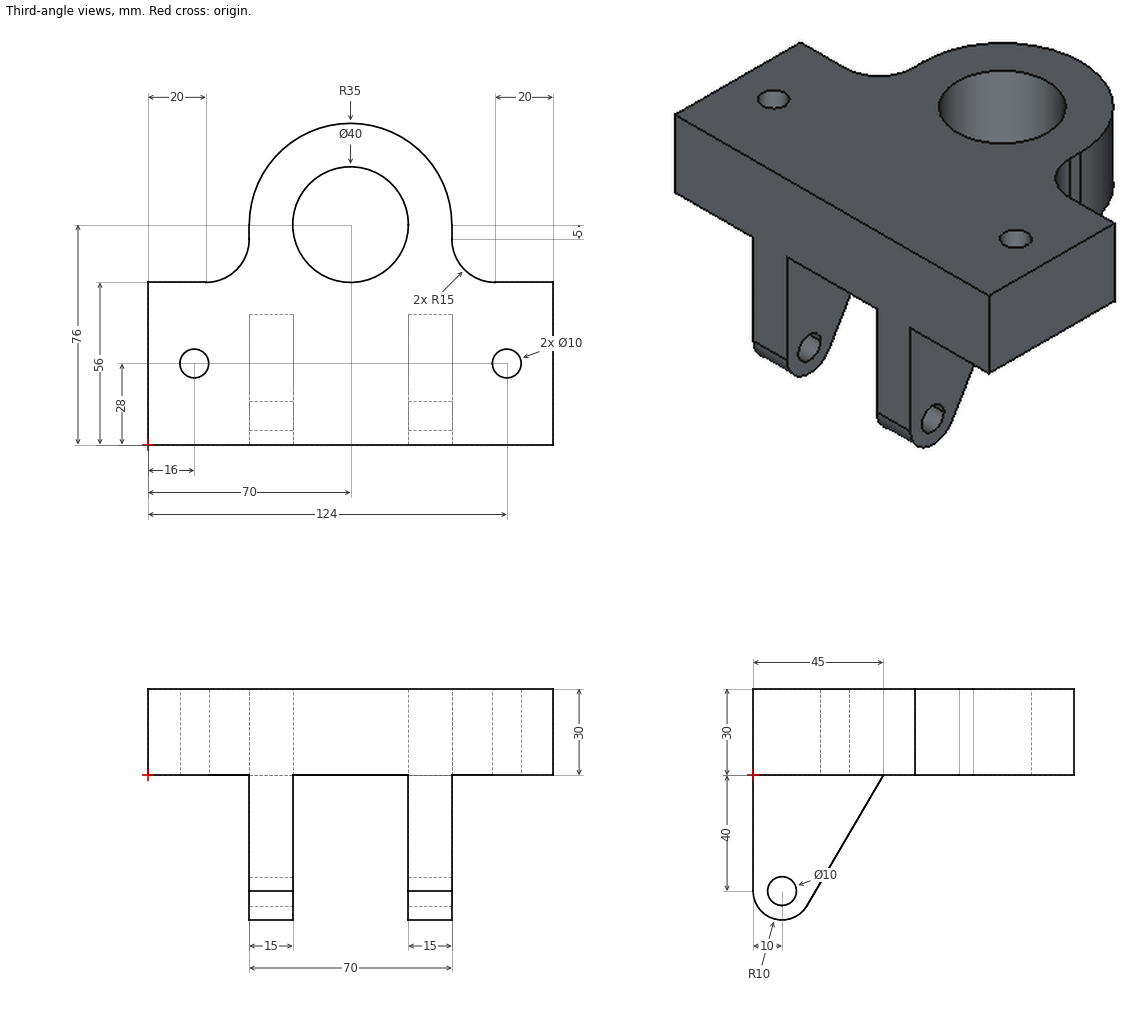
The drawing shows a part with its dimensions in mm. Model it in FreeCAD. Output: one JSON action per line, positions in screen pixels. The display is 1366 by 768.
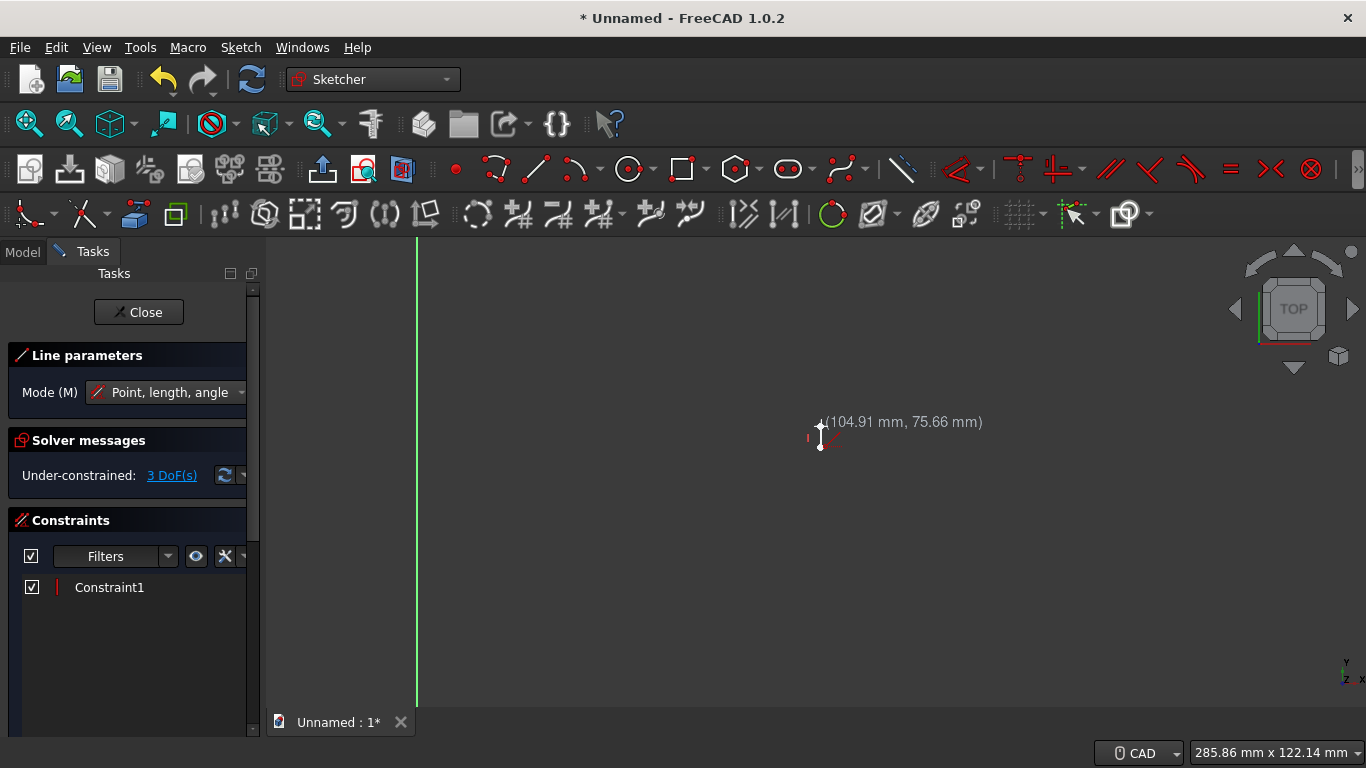
{"action": "left_click", "coordinate": [552, 426]}
{"action": "left_click", "coordinate": [552, 445]}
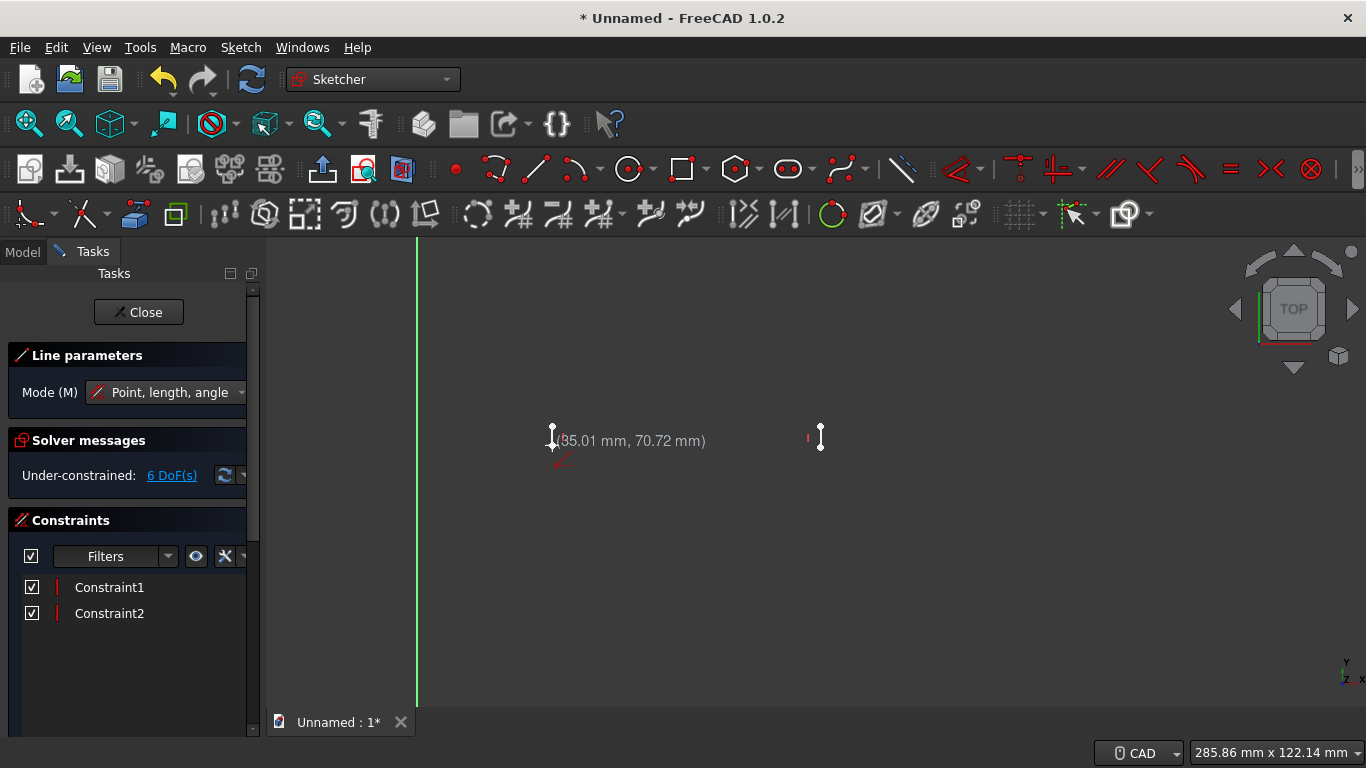
{"action": "left_click", "coordinate": [496, 170]}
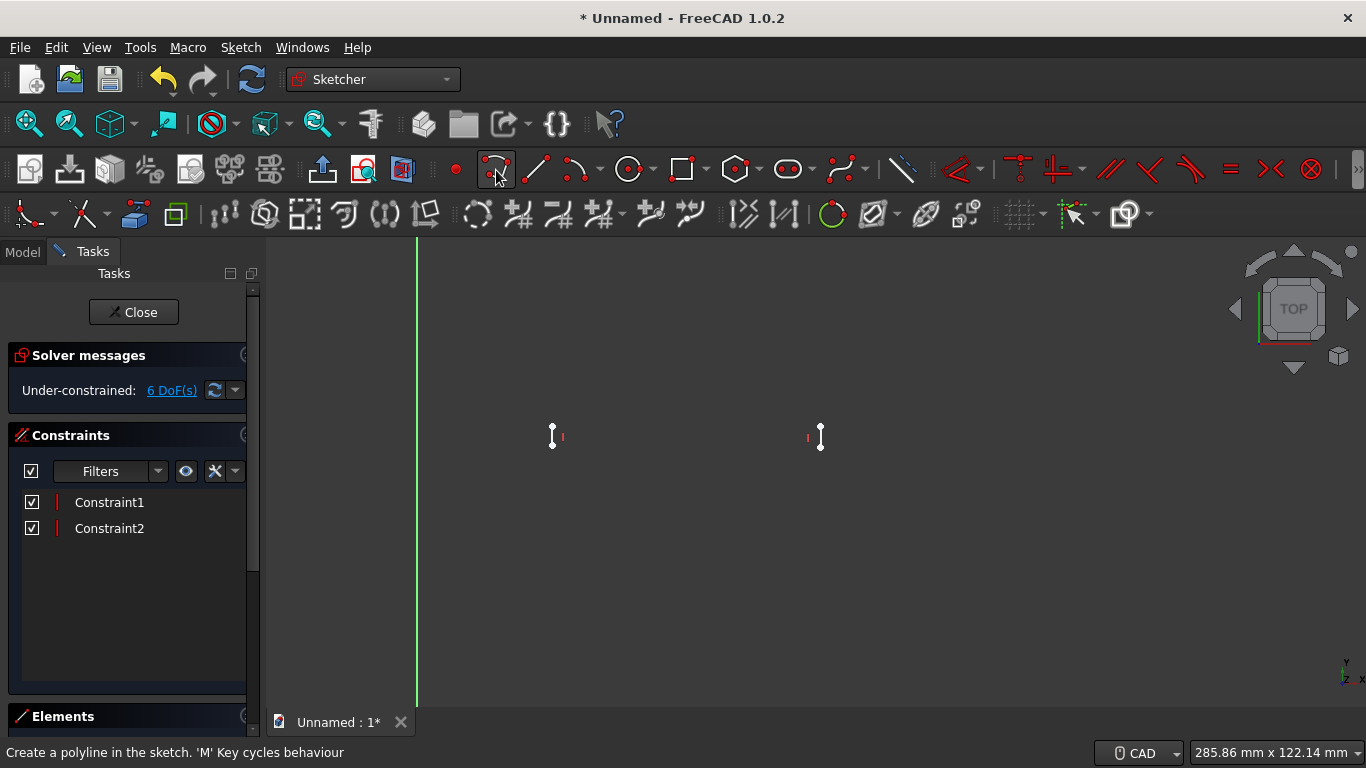
{"action": "left_click", "coordinate": [494, 503]}
{"action": "left_click", "coordinate": [417, 503]}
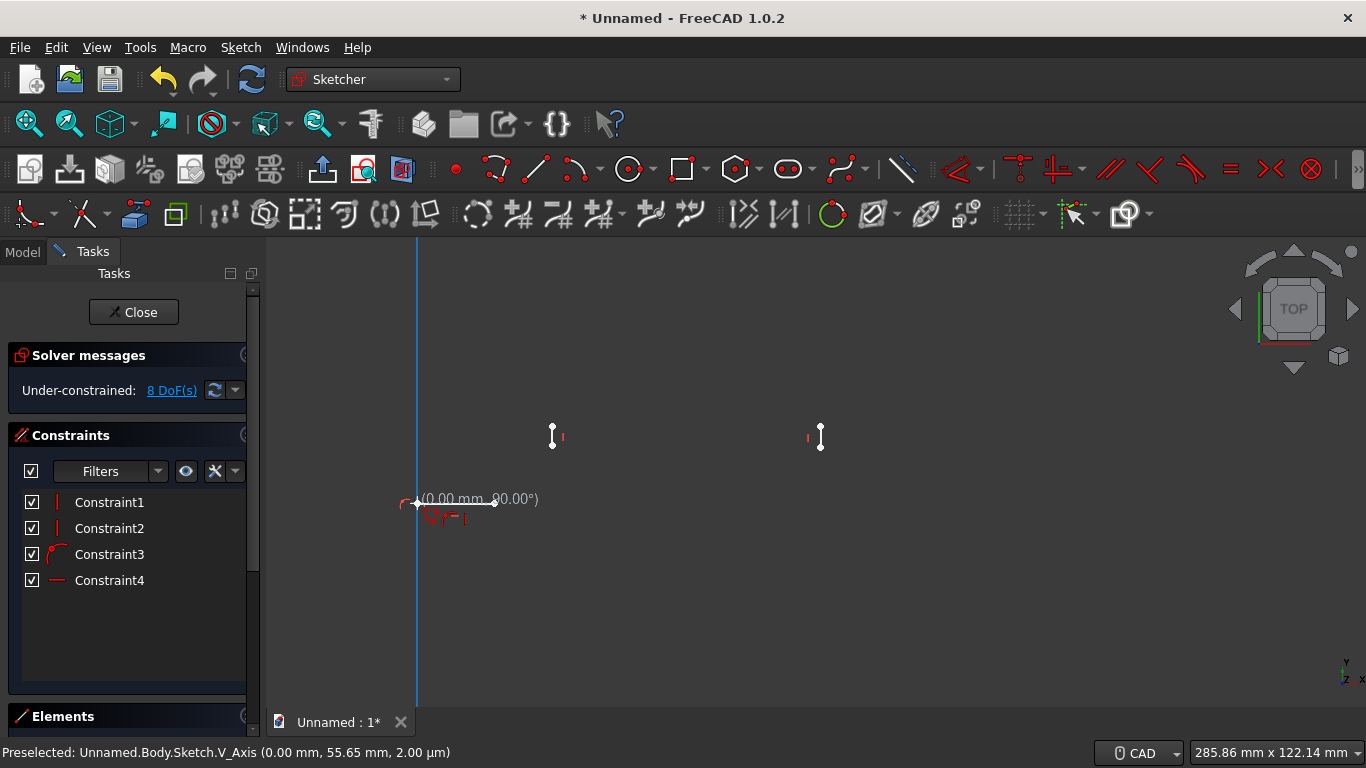
{"action": "scroll", "coordinate": [871, 406], "scroll_direction": "down", "scroll_amount": 2}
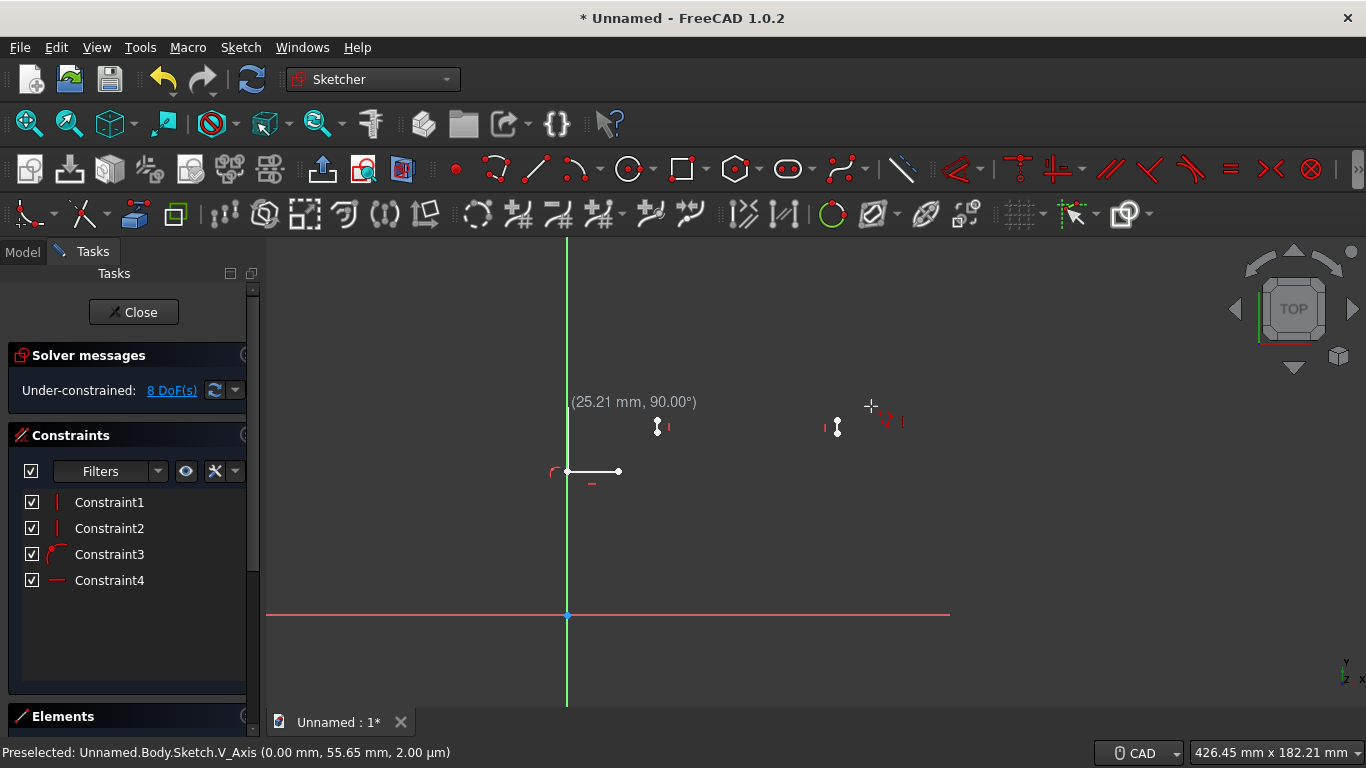
{"action": "left_click", "coordinate": [567, 615]}
{"action": "left_click", "coordinate": [928, 606]}
{"action": "left_click", "coordinate": [928, 471]}
{"action": "left_click", "coordinate": [877, 471]}
{"action": "right_click", "coordinate": [877, 471]}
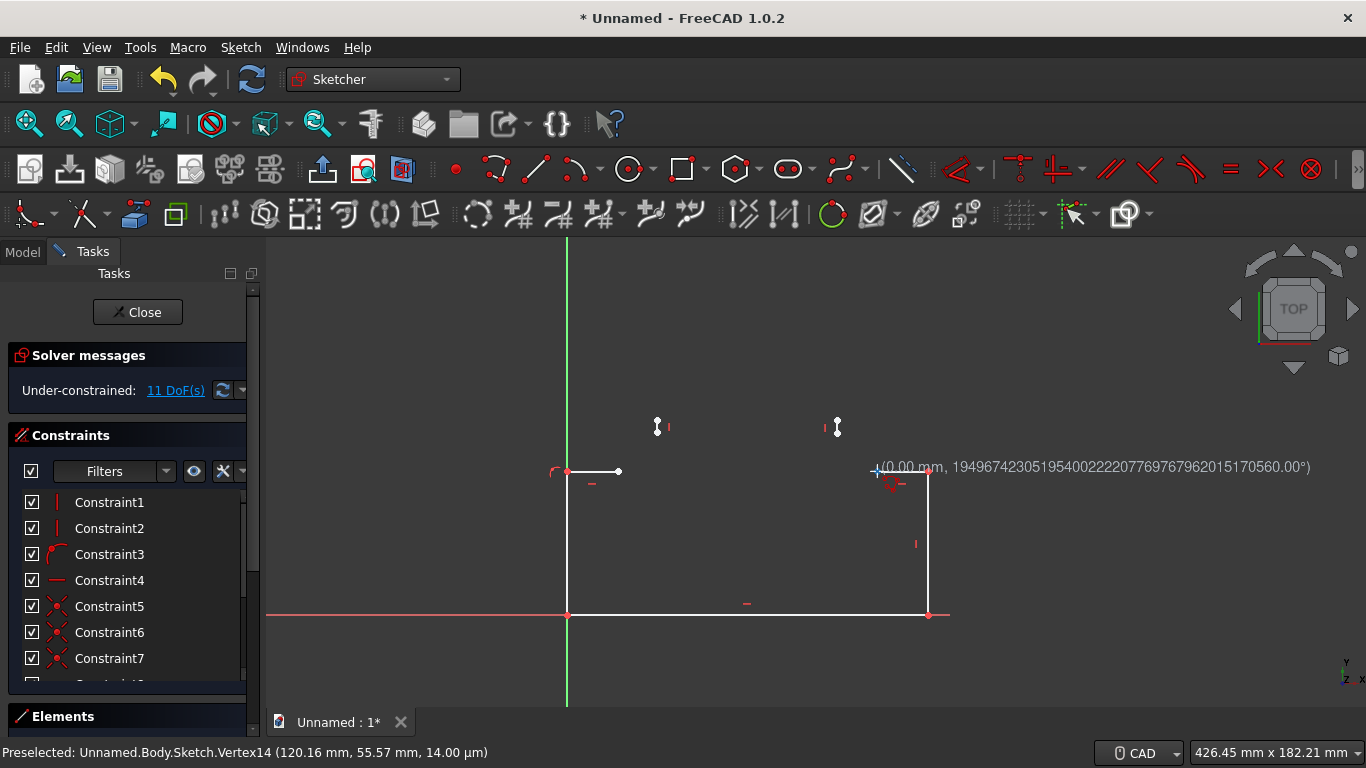
{"action": "key", "text": "g 3 a"}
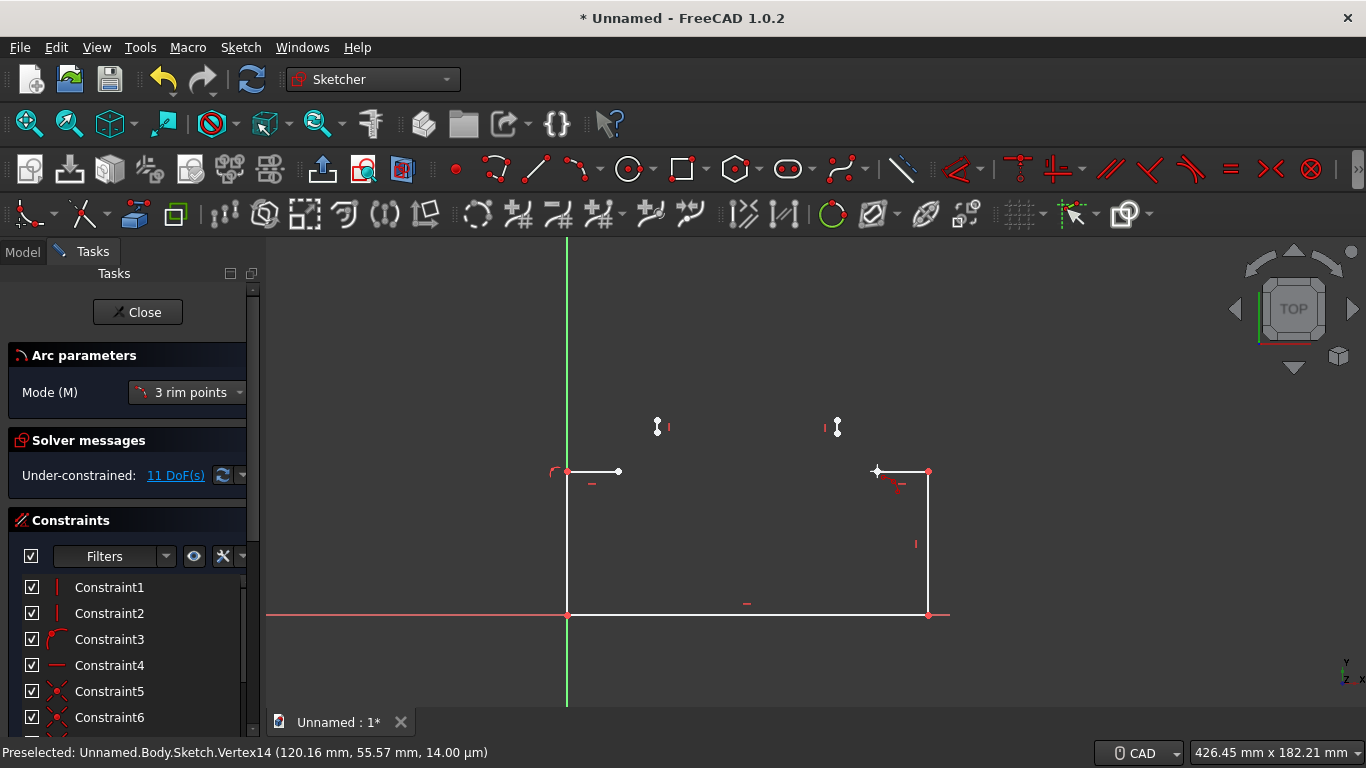
{"action": "scroll", "coordinate": [838, 419], "scroll_direction": "up", "scroll_amount": 5}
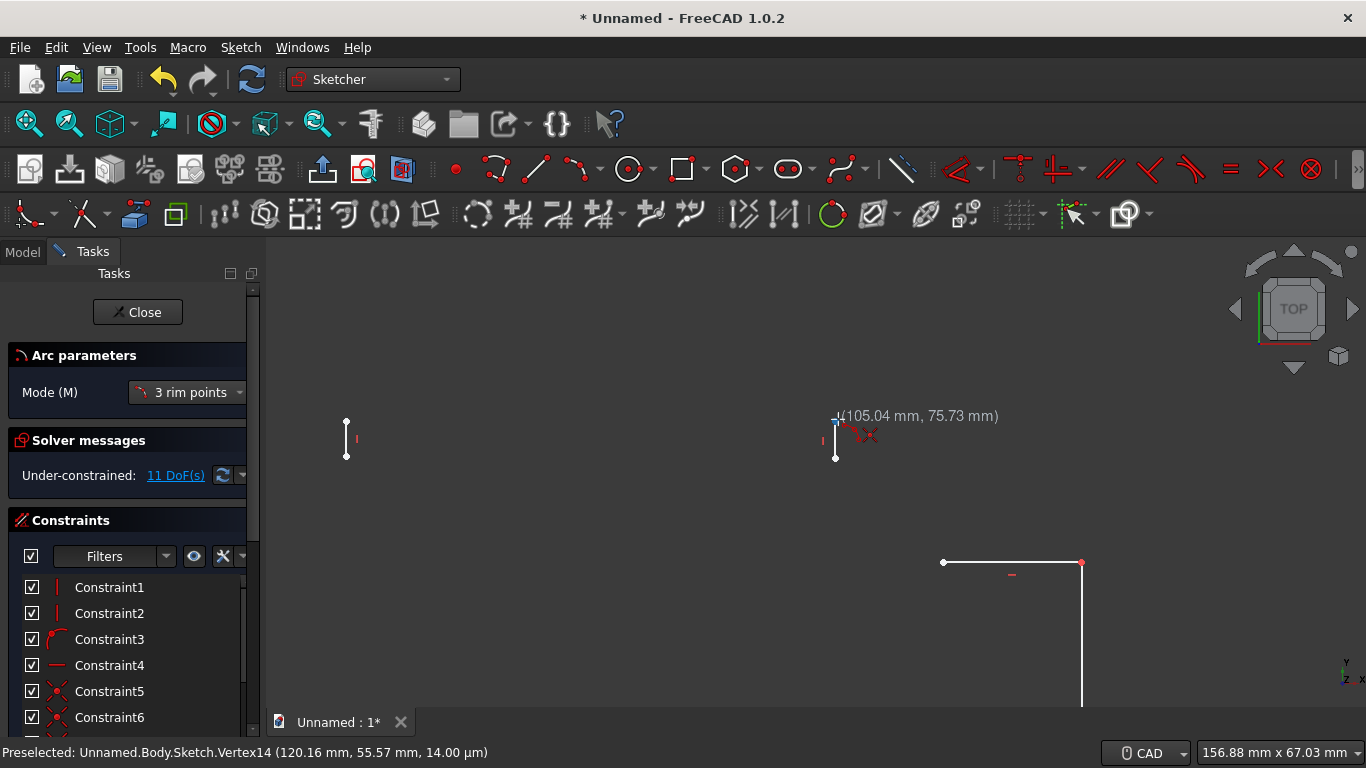
{"action": "left_click", "coordinate": [835, 422]}
{"action": "left_click", "coordinate": [346, 422]}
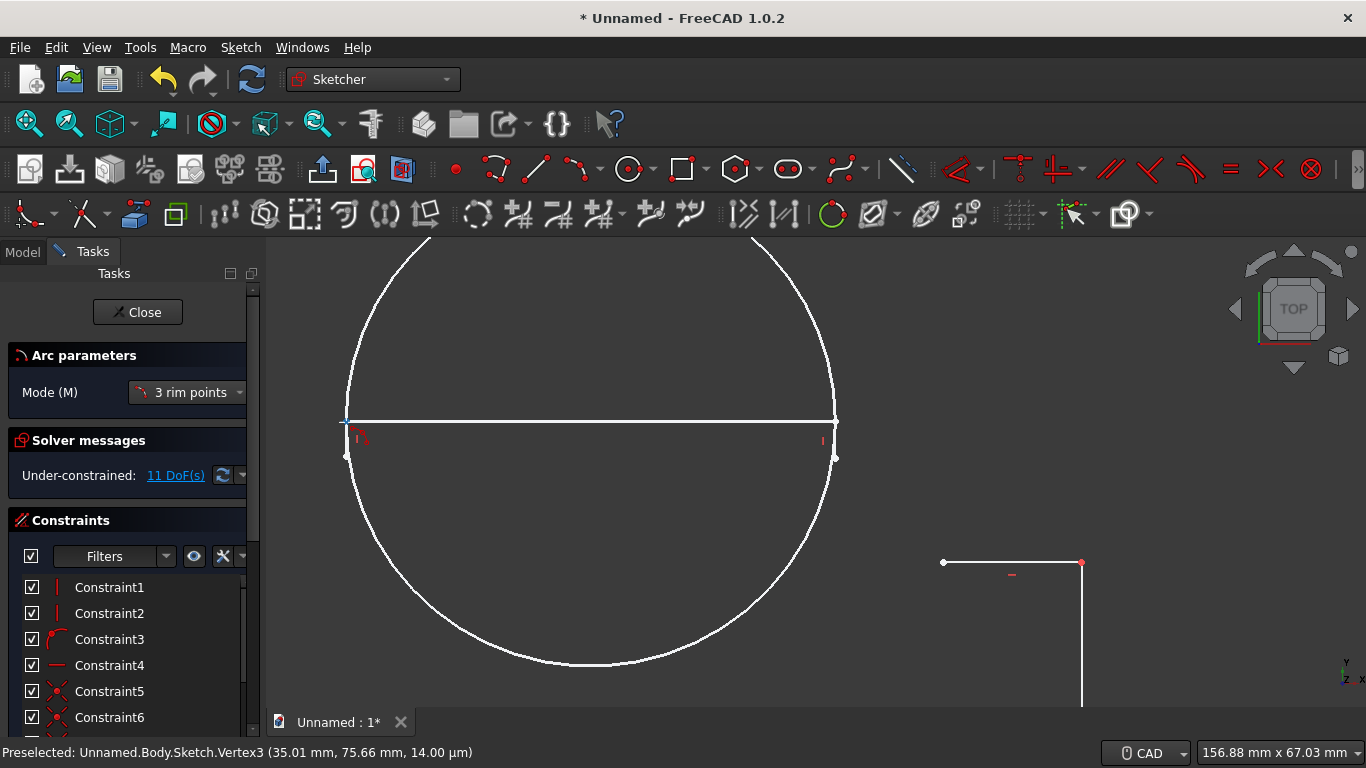
{"action": "scroll", "coordinate": [838, 419], "scroll_direction": "down", "scroll_amount": 5}